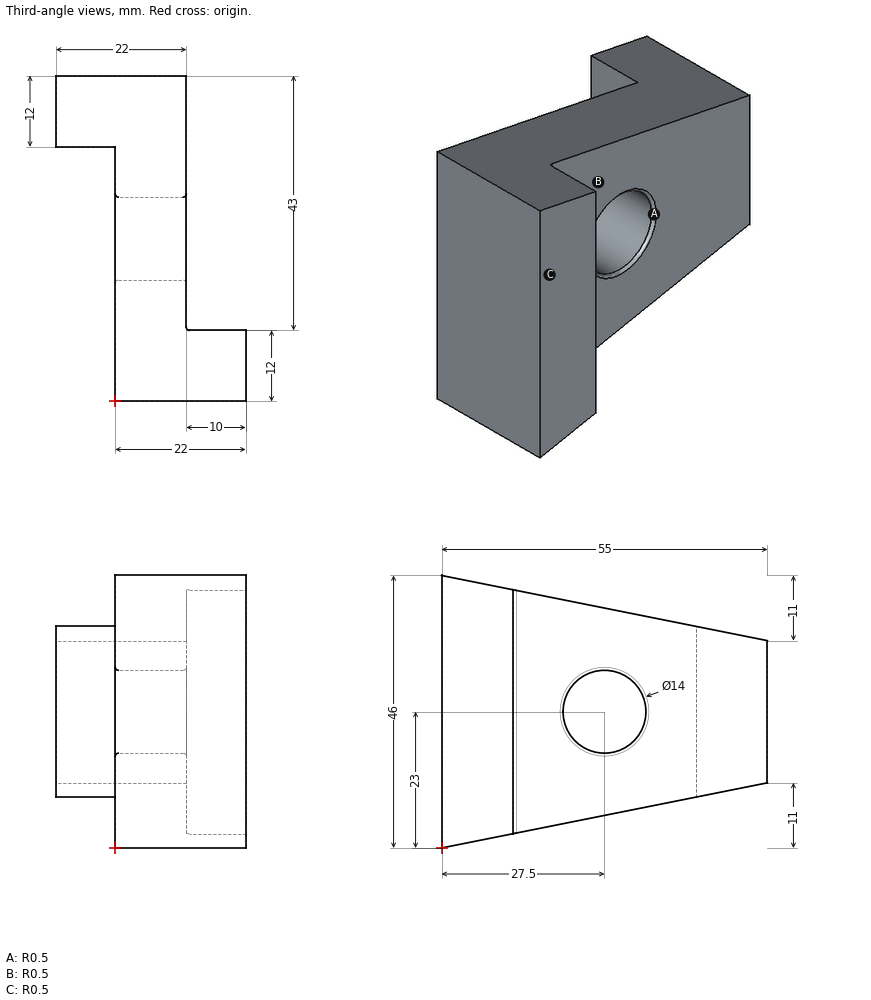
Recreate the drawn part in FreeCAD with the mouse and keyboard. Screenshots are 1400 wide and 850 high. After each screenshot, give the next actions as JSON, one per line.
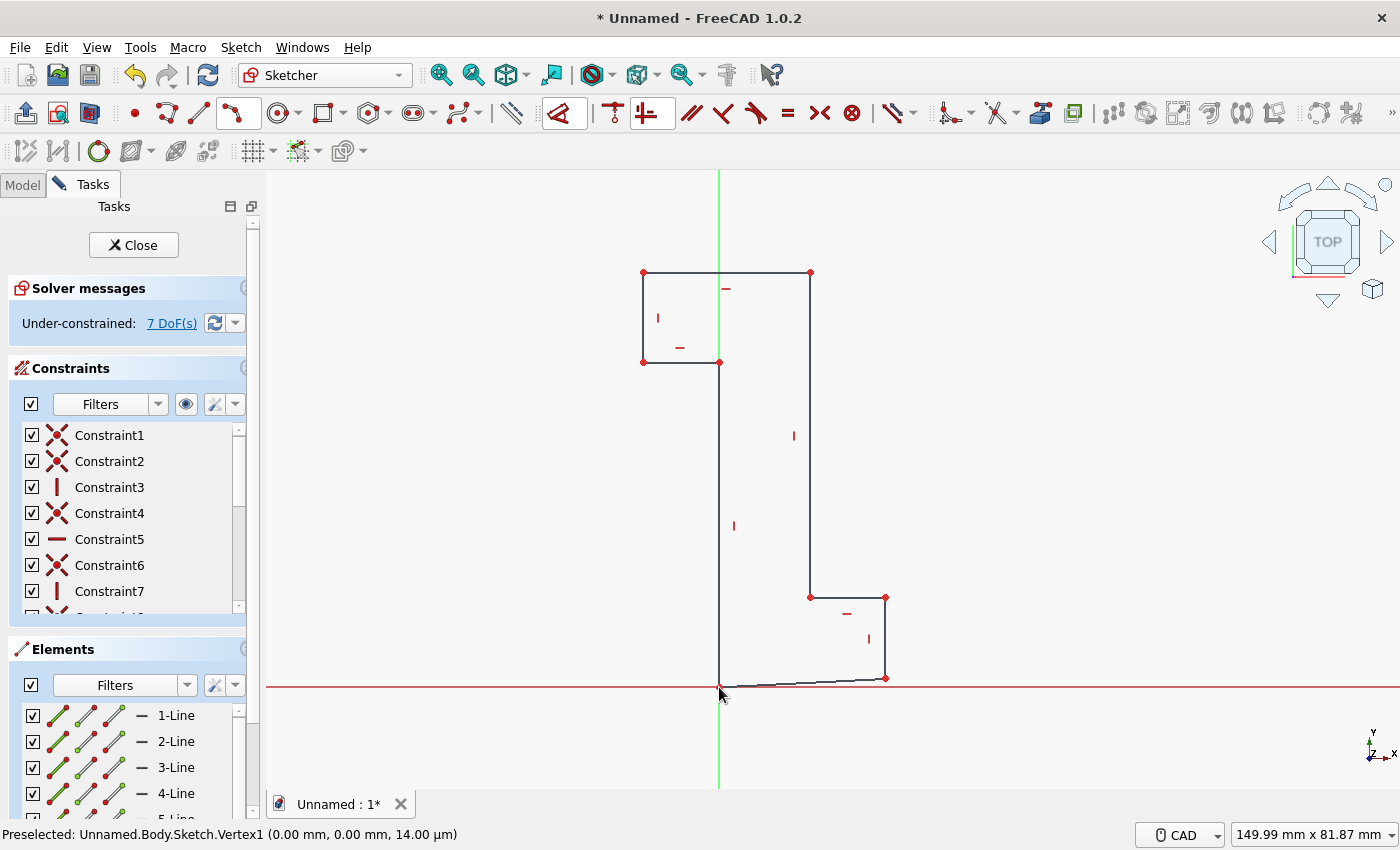
{"action": "left_click", "coordinate": [769, 685]}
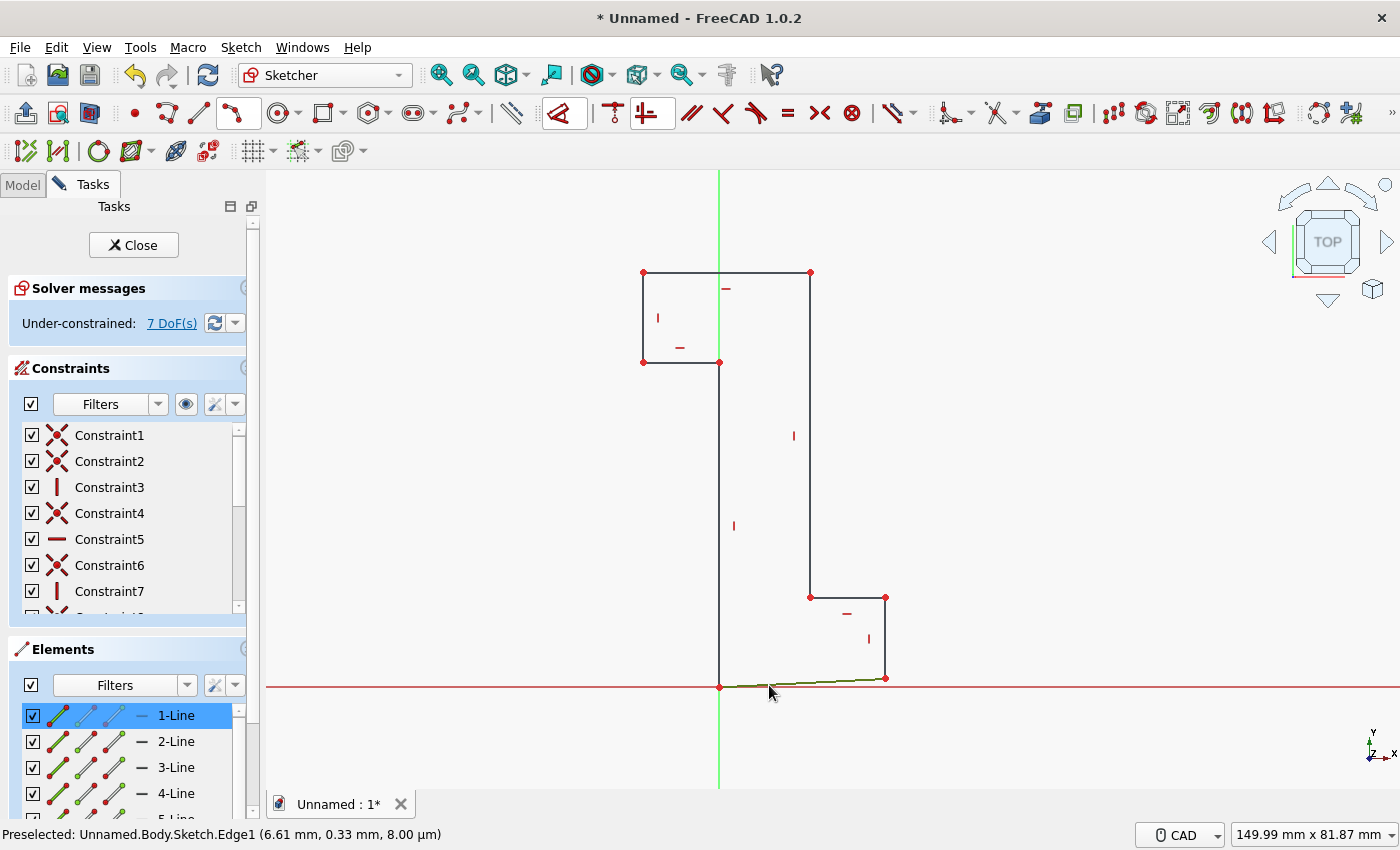
{"action": "key", "text": "h"}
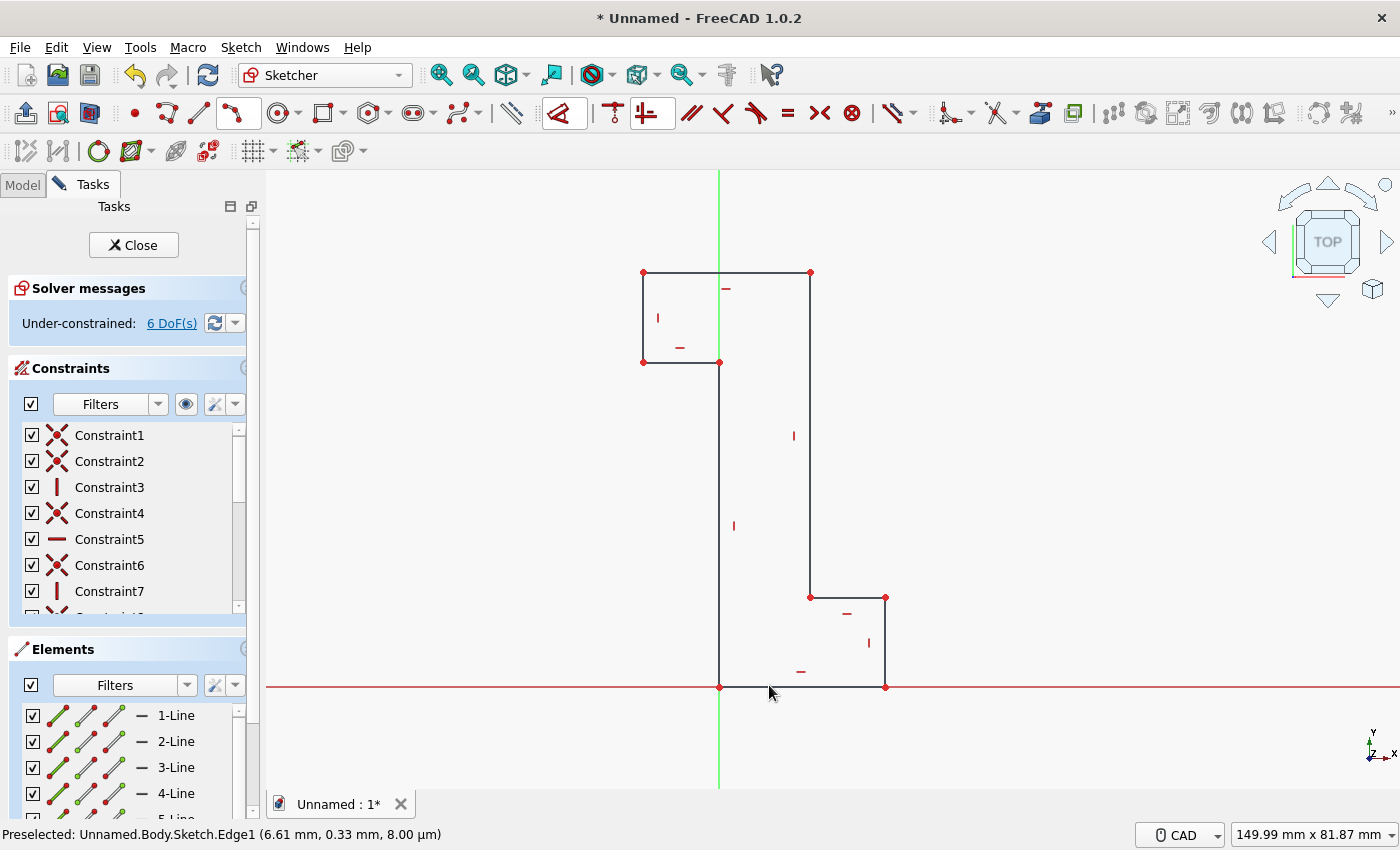
{"action": "left_click", "coordinate": [769, 687]}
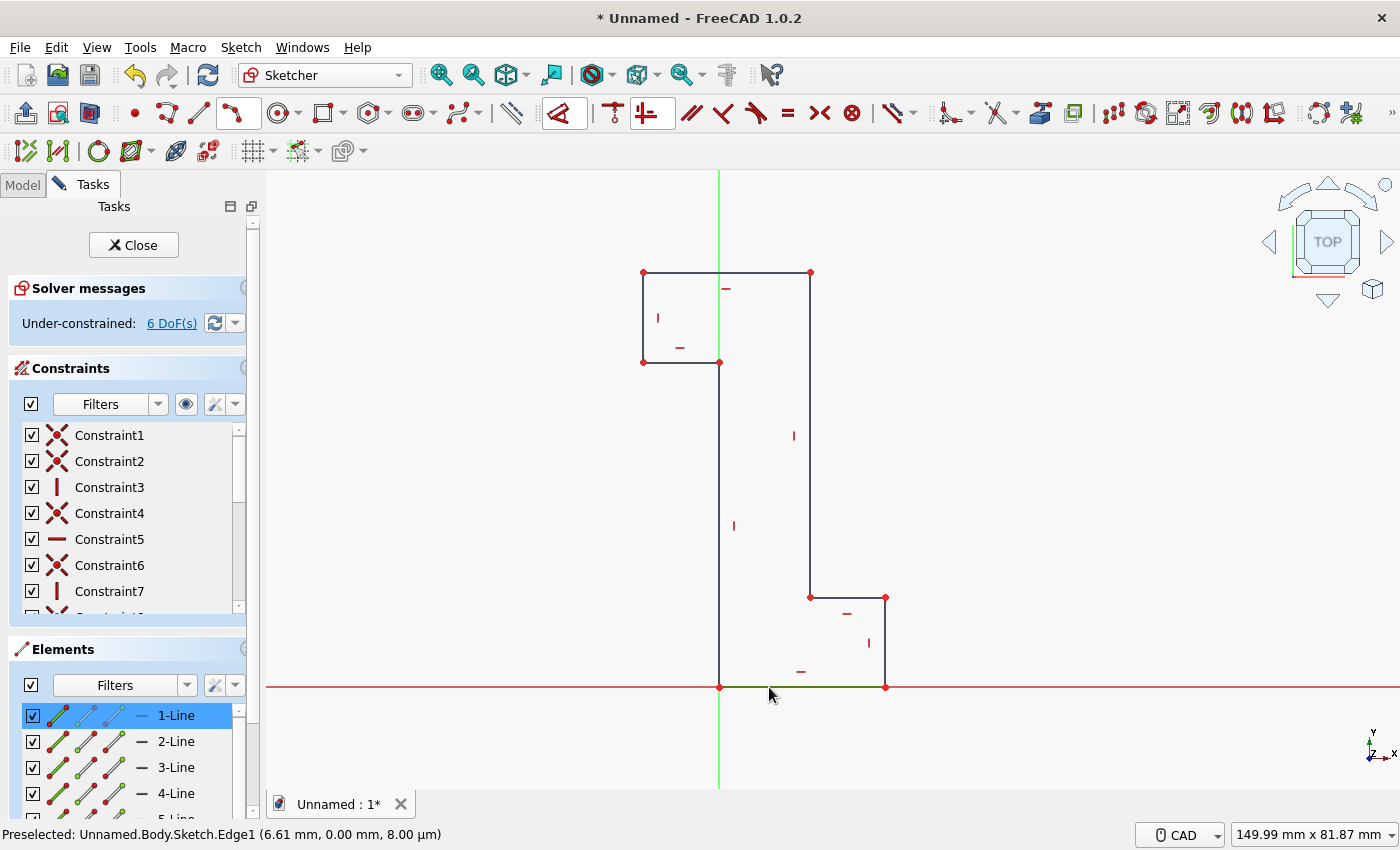
{"action": "key", "text": "l"}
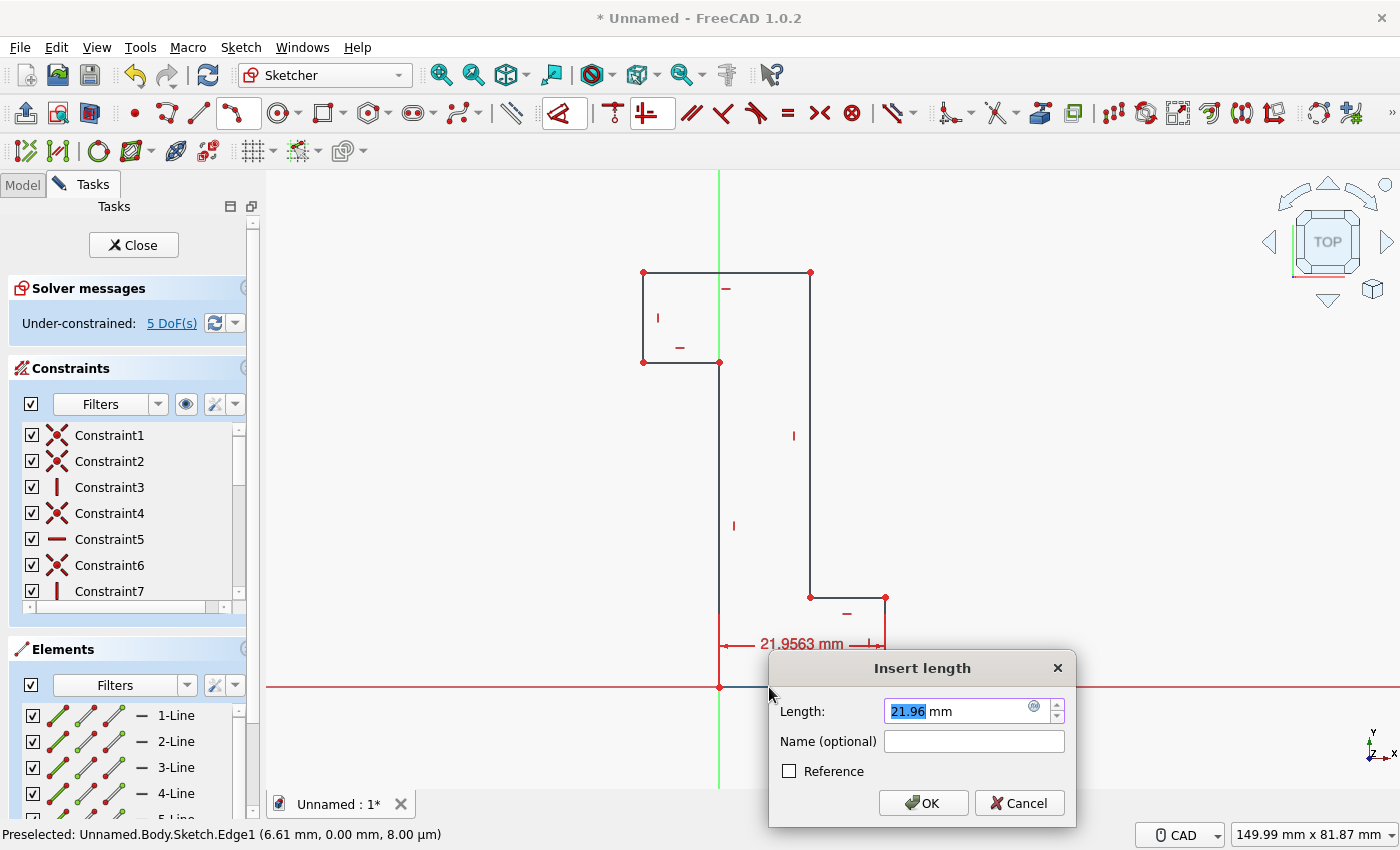
{"action": "type", "text": "22"}
{"action": "key", "text": "Return"}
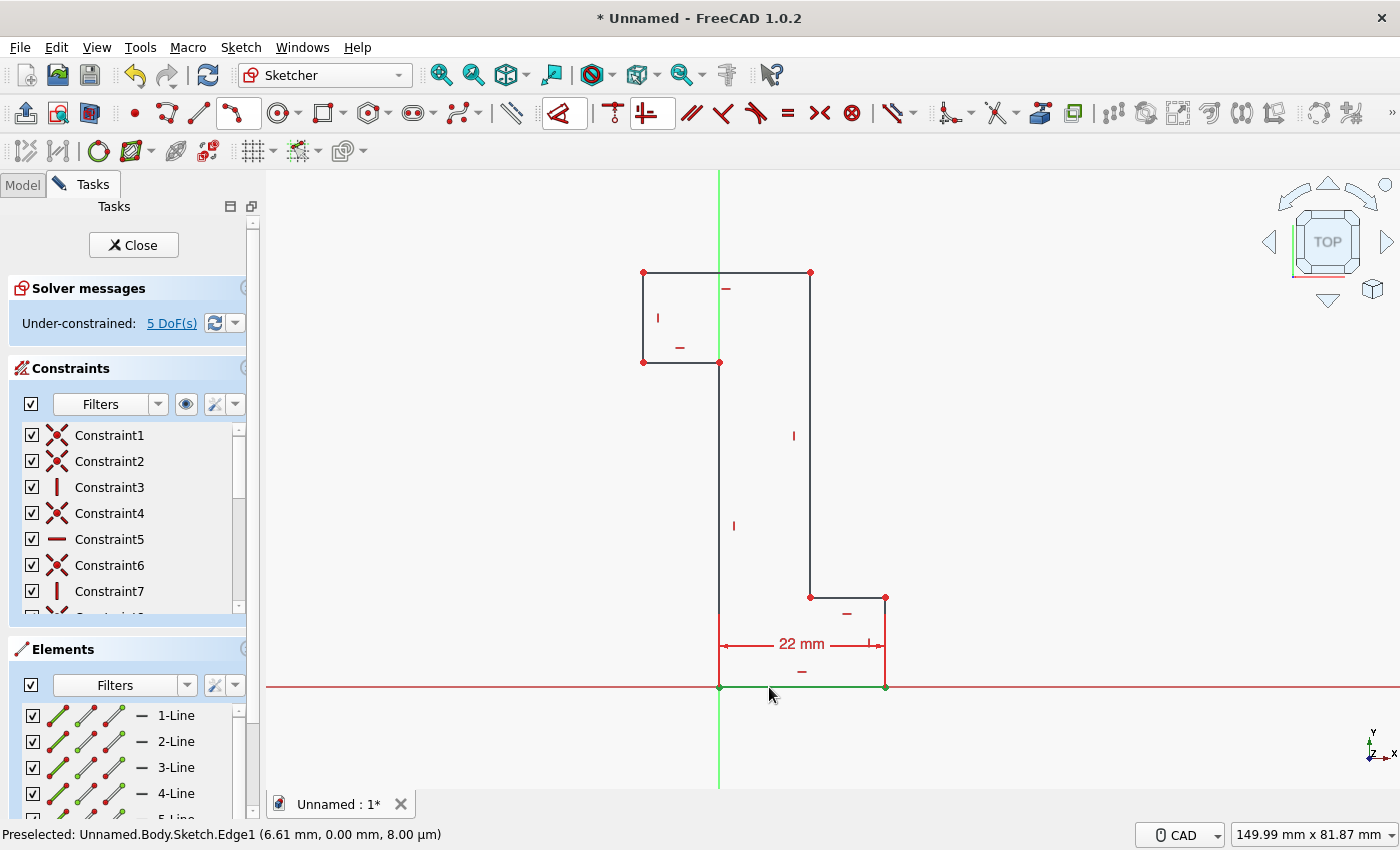
{"action": "left_click", "coordinate": [885, 661]}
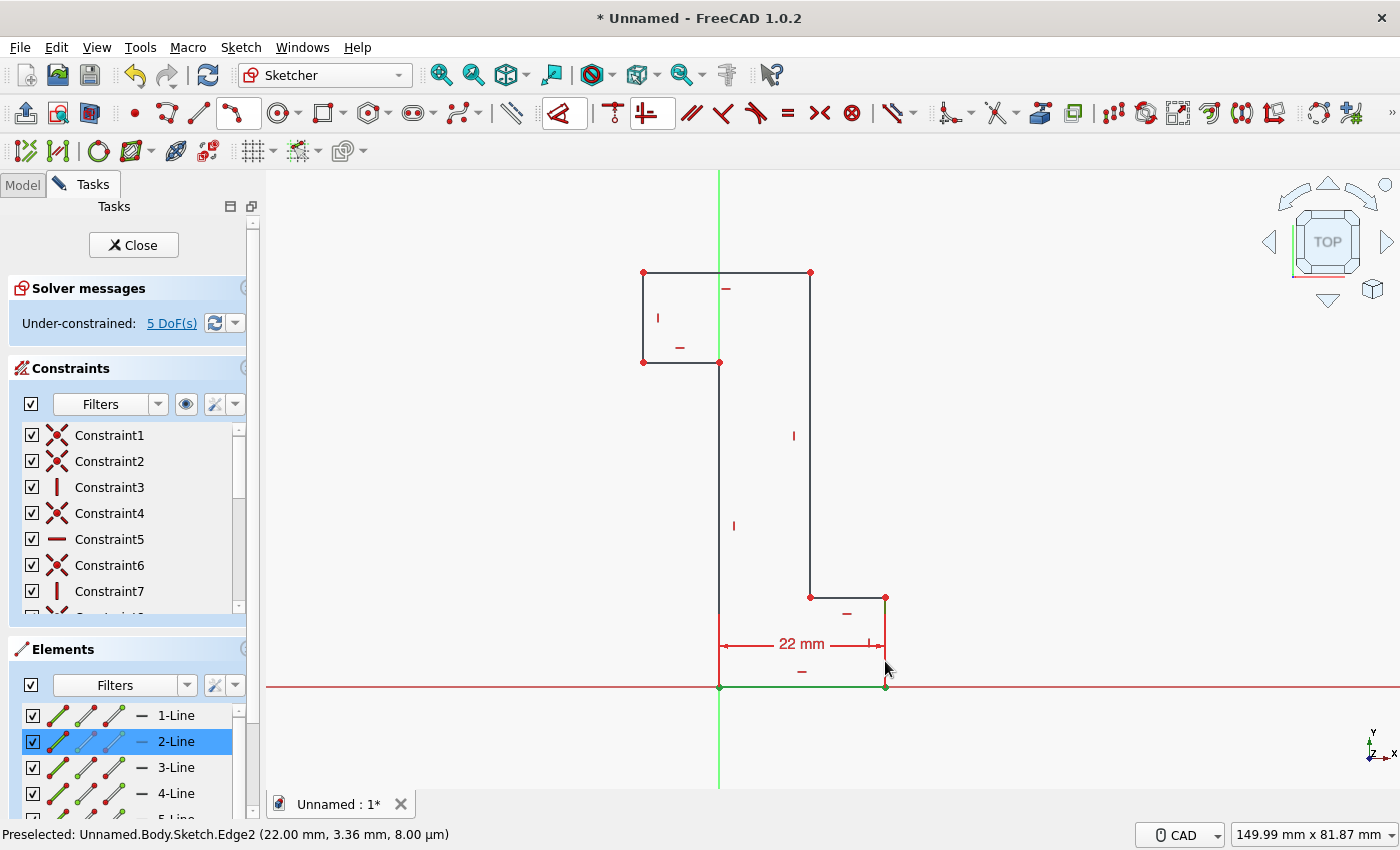
{"action": "key", "text": "i"}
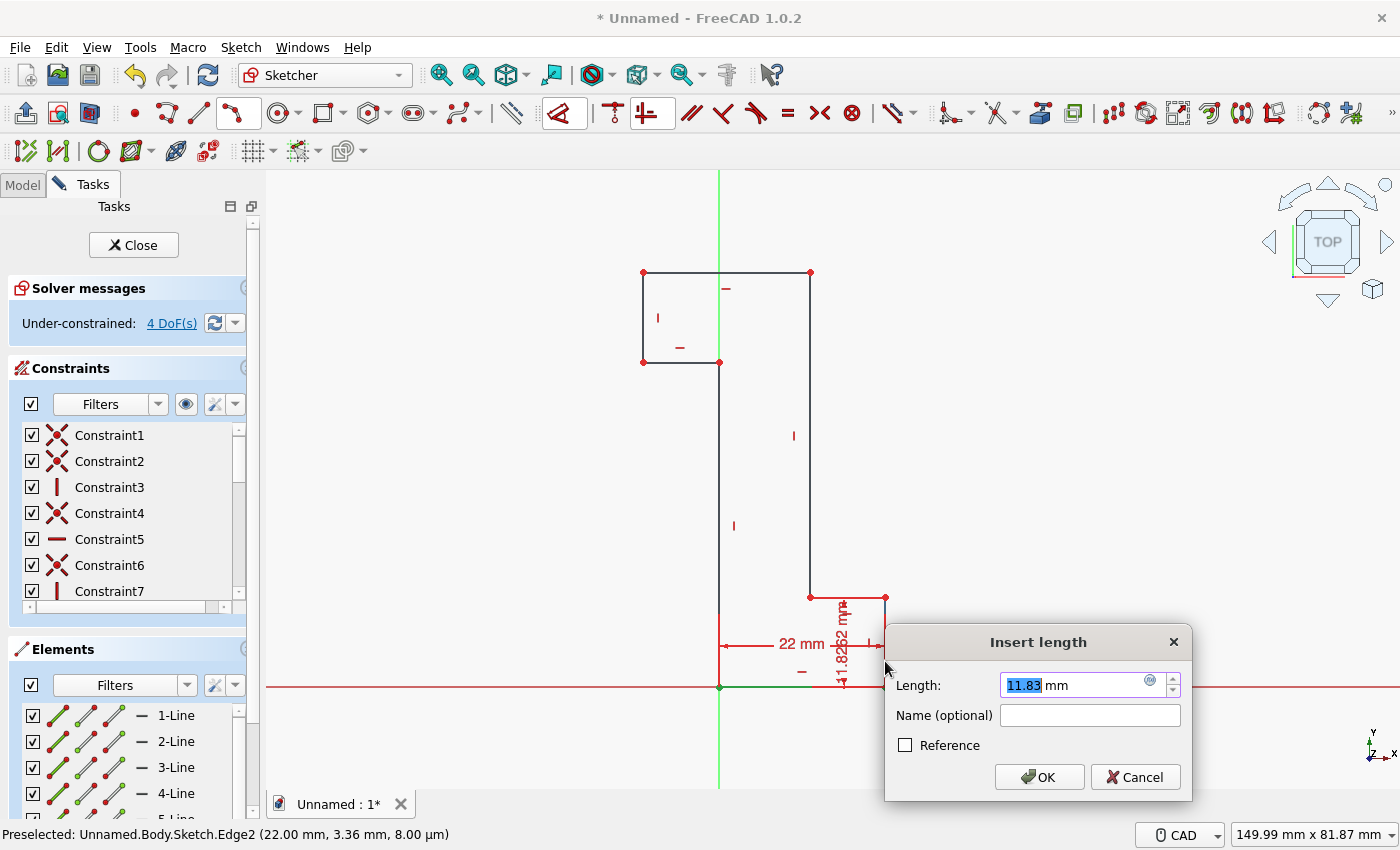
{"action": "type", "text": "12"}
{"action": "key", "text": "Return"}